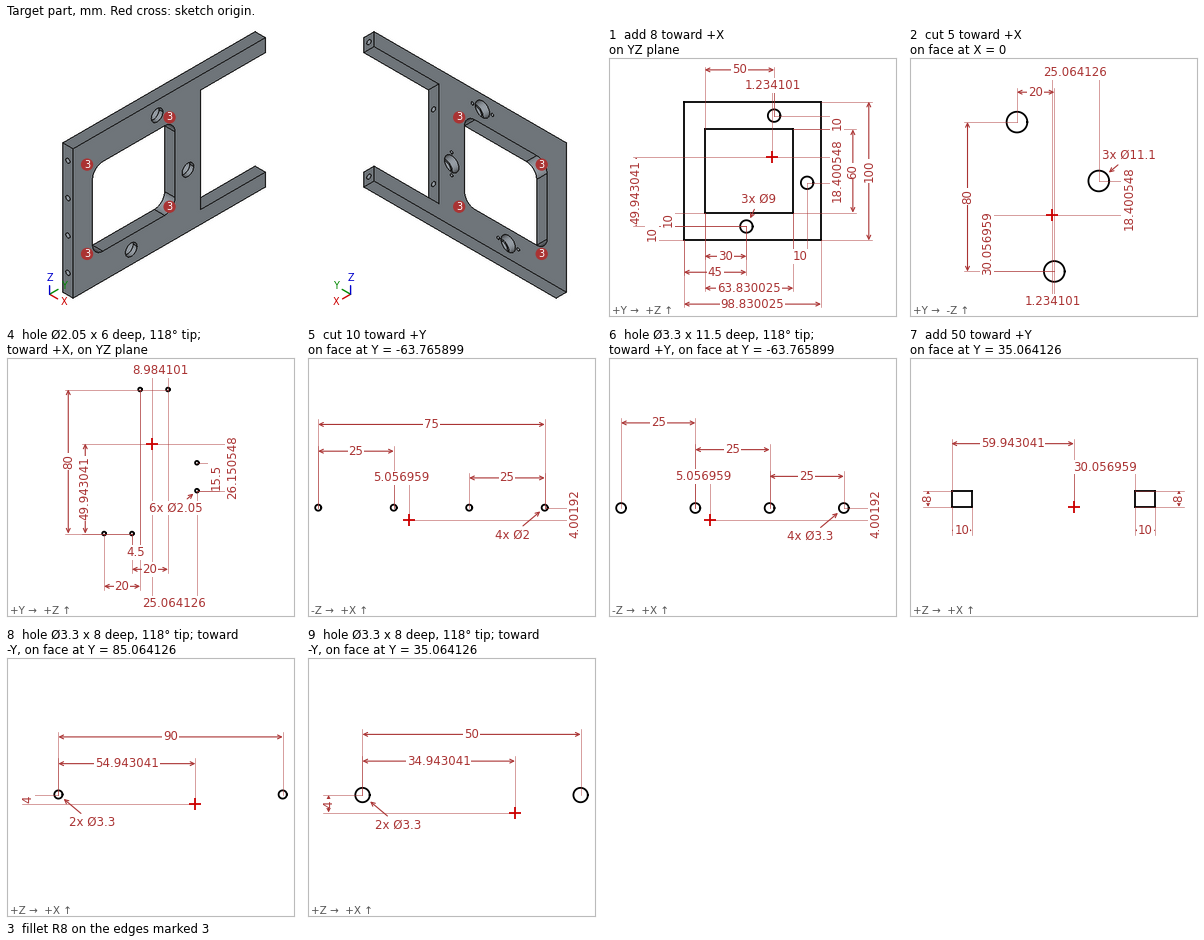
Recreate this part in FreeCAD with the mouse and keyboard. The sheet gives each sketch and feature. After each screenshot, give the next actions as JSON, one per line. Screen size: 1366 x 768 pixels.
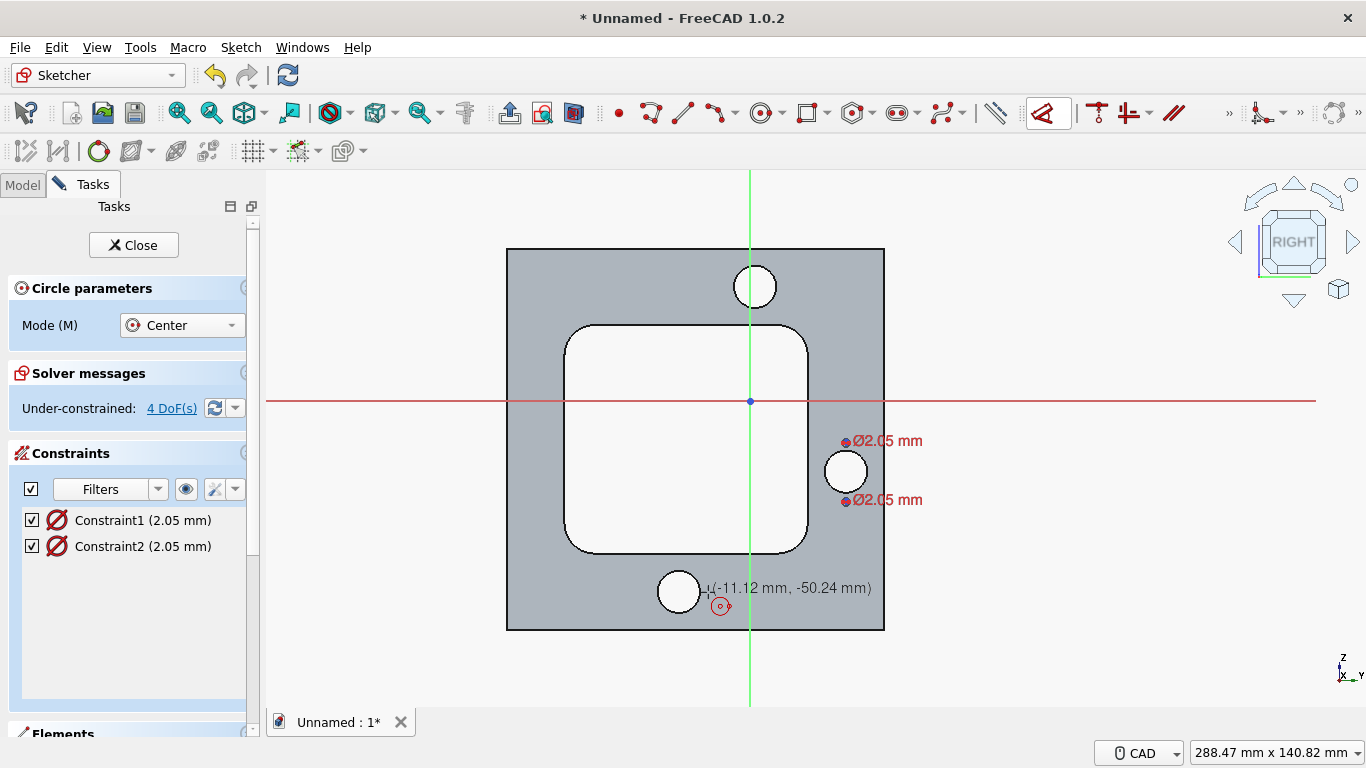
{"action": "left_click", "coordinate": [708, 592]}
{"action": "mouse_move", "coordinate": [711, 589]}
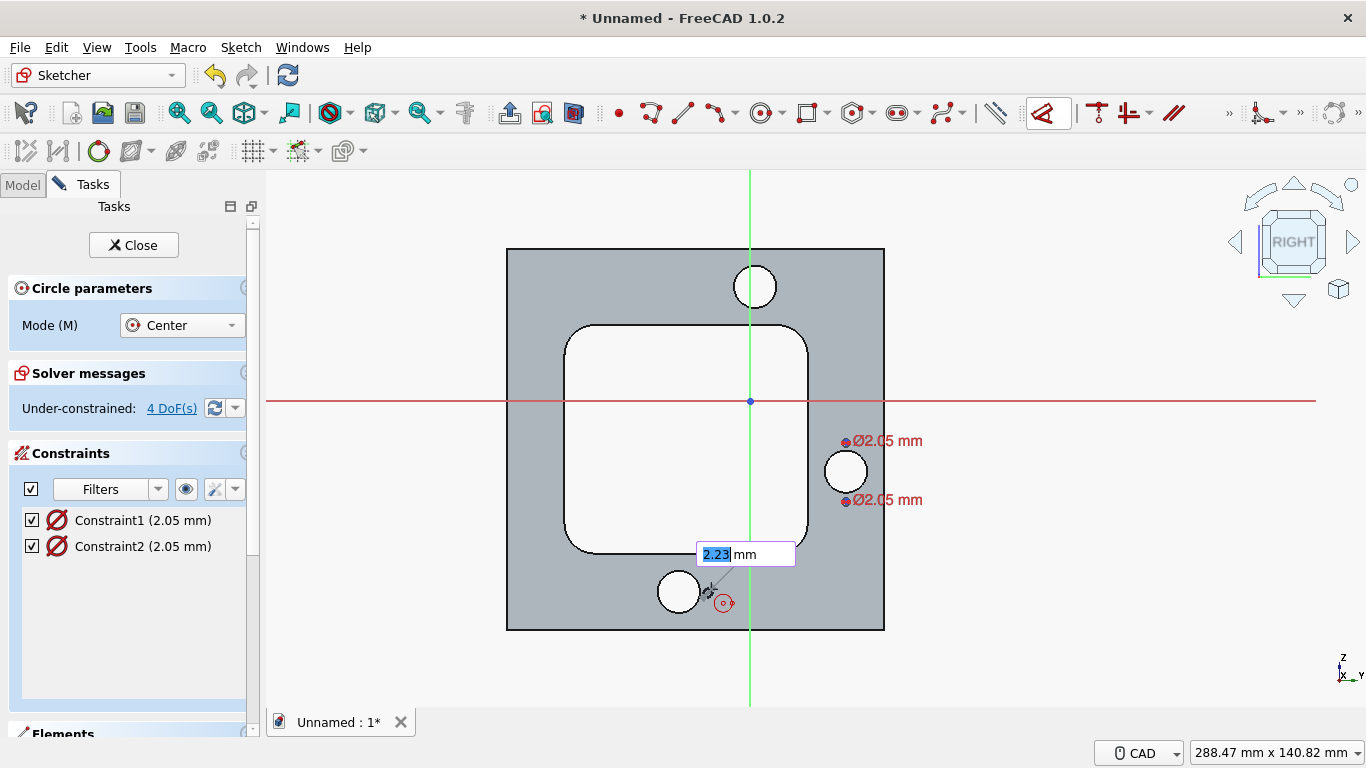
{"action": "type", "text": "2.05"}
{"action": "key", "text": "Return"}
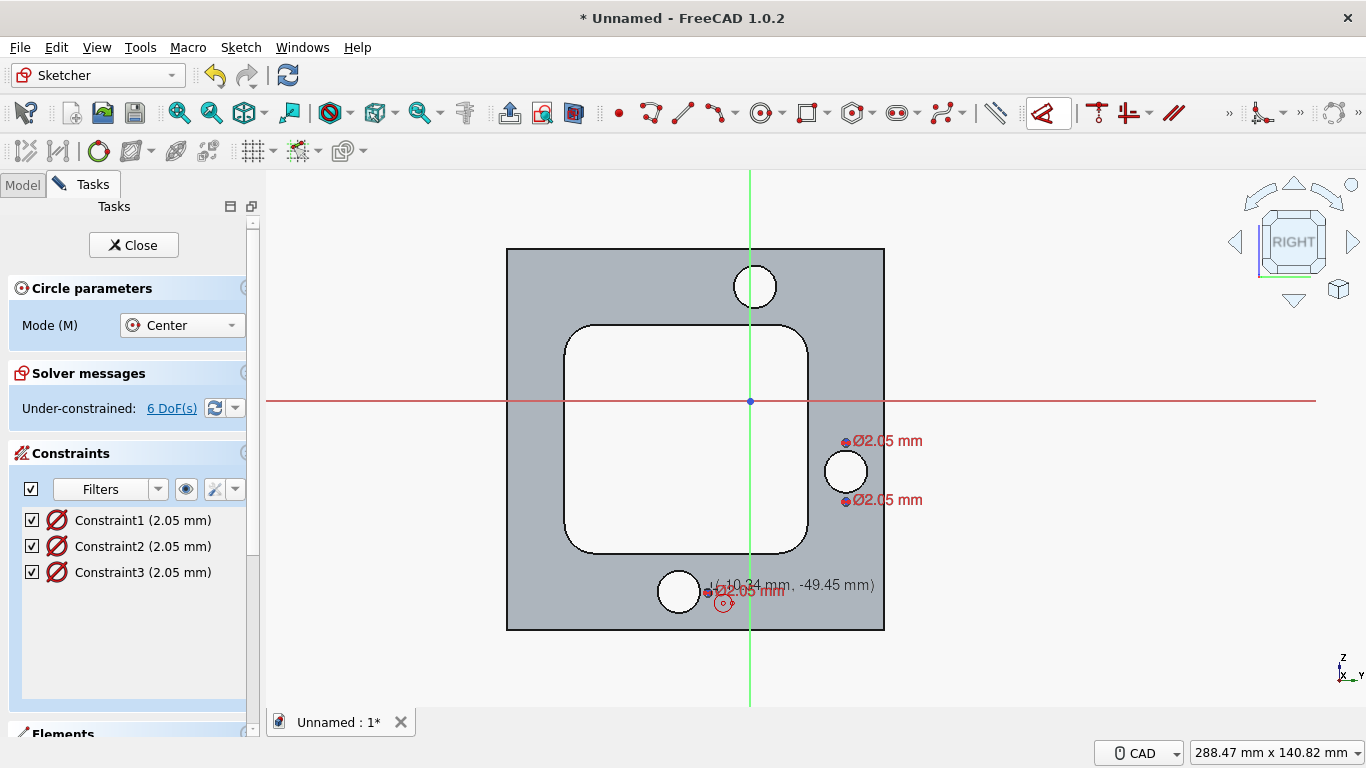
{"action": "scroll", "coordinate": [649, 592], "scroll_direction": "up", "scroll_amount": 9}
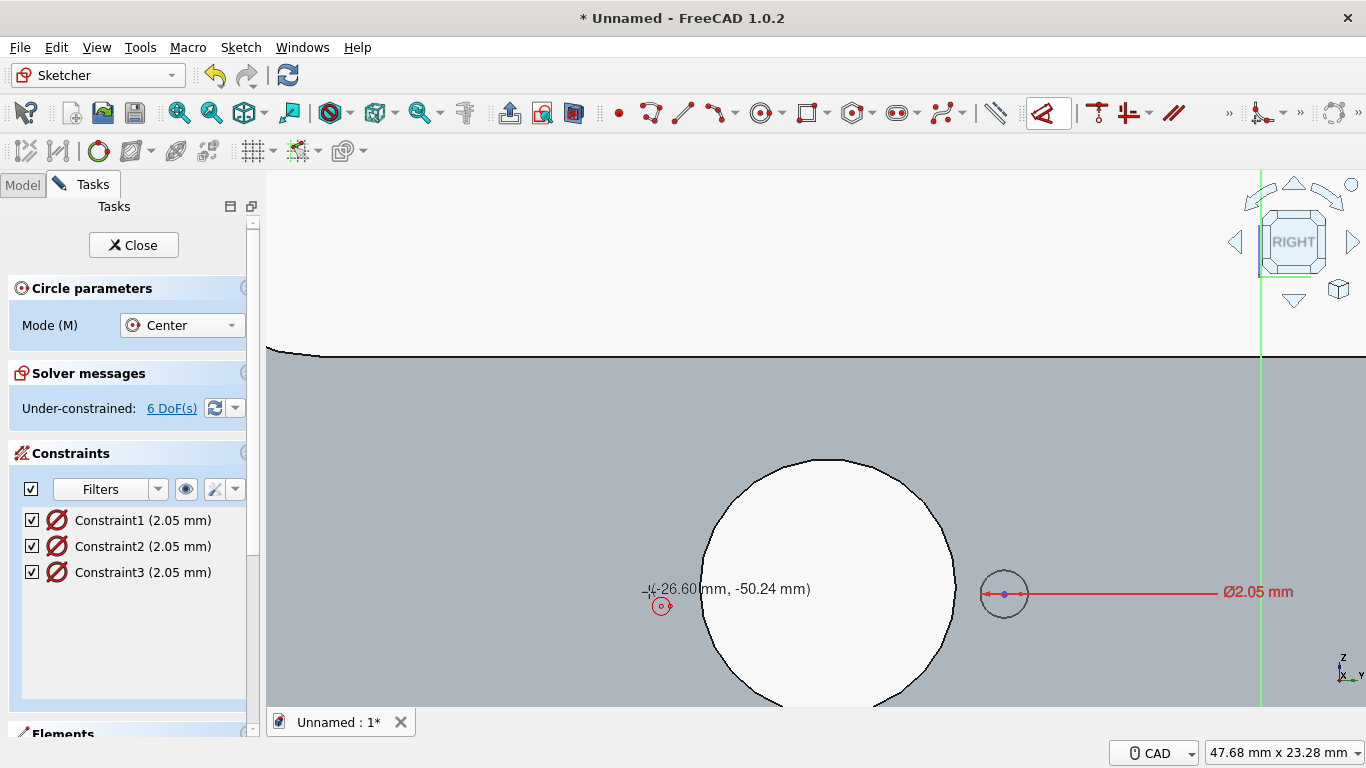
{"action": "scroll", "coordinate": [649, 592], "scroll_direction": "down", "scroll_amount": 9}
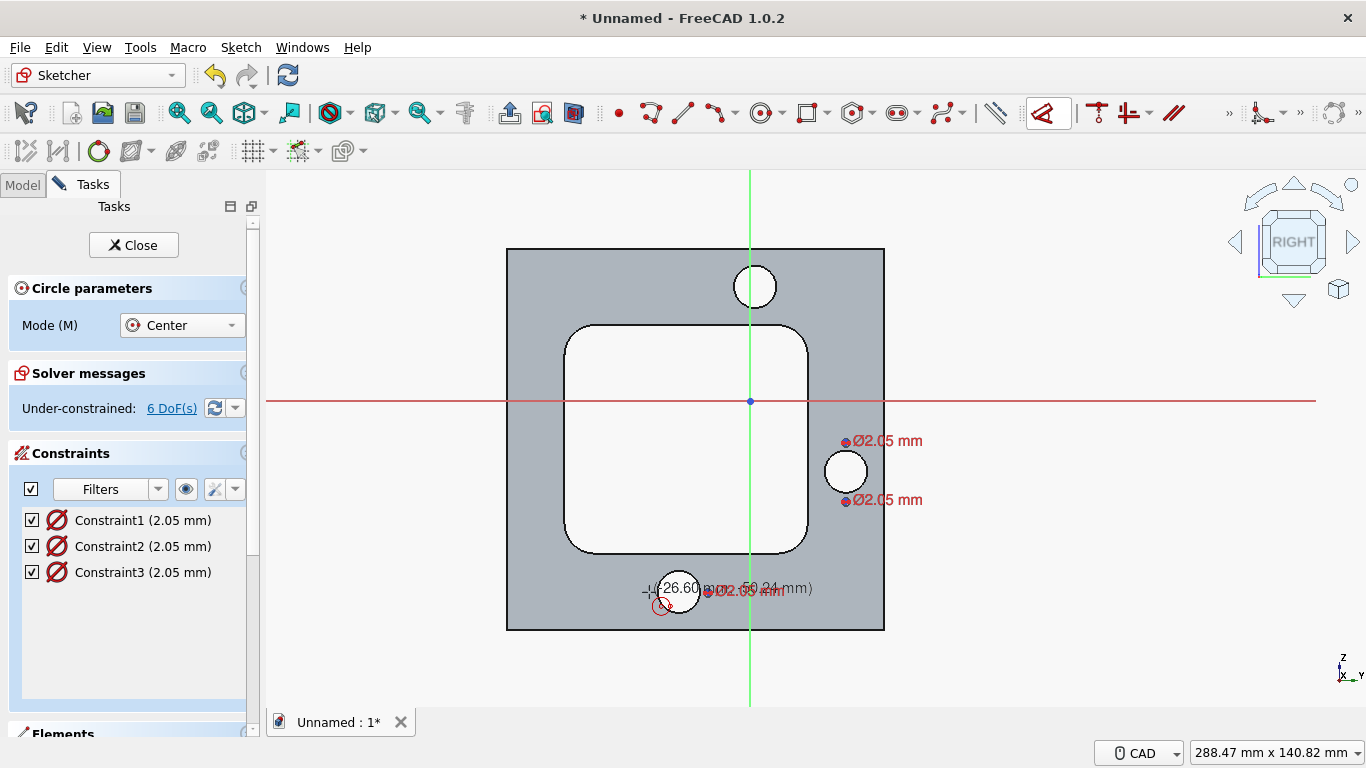
{"action": "left_click", "coordinate": [649, 592]}
{"action": "mouse_move", "coordinate": [652, 589]}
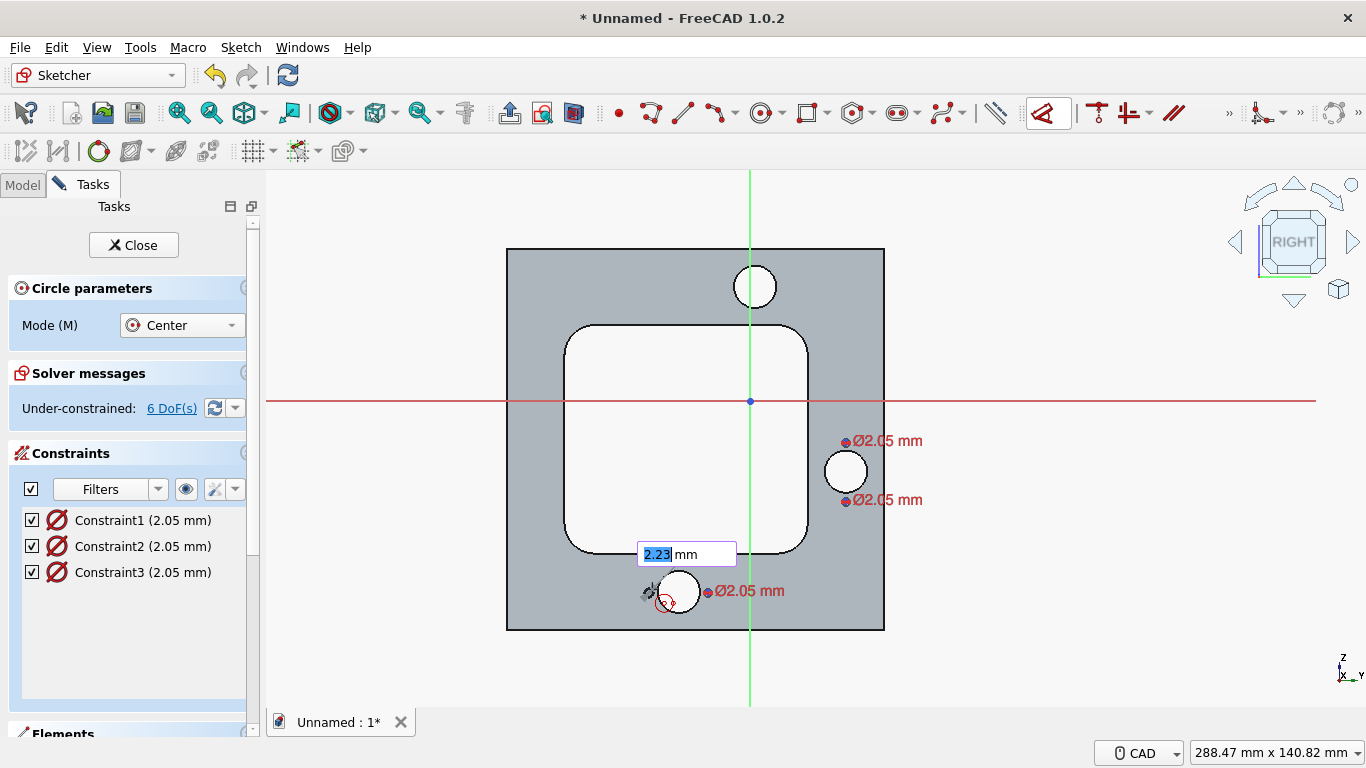
{"action": "type", "text": "2.05"}
{"action": "key", "text": "Return"}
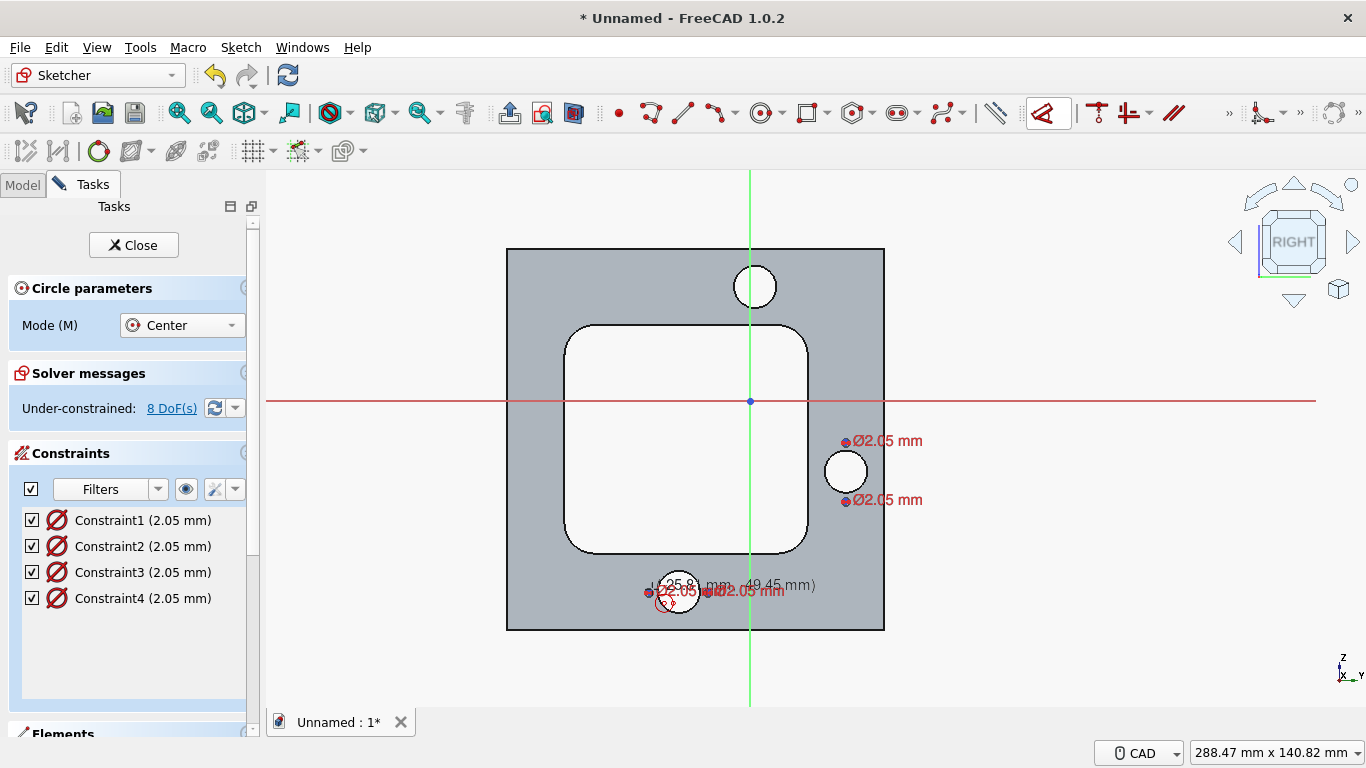
{"action": "scroll", "coordinate": [785, 287], "scroll_direction": "up", "scroll_amount": 9}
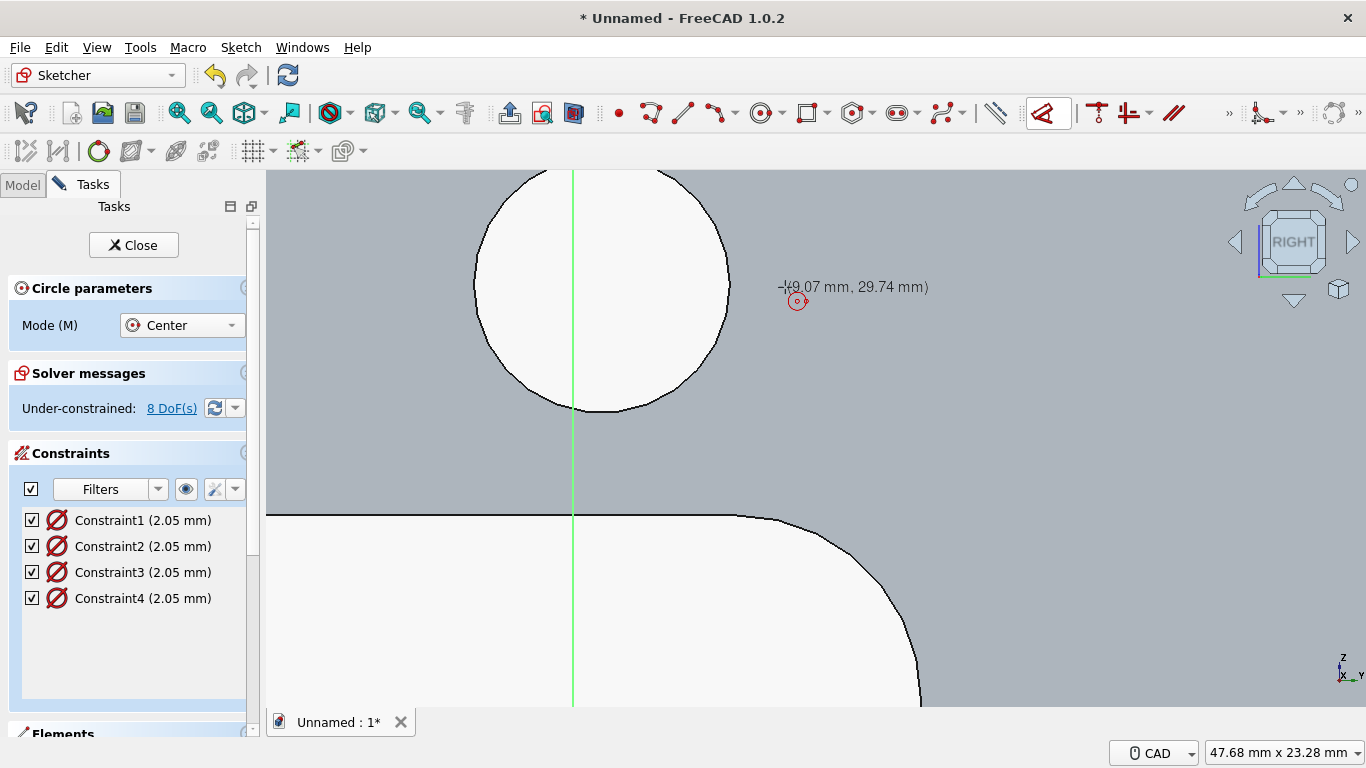
{"action": "scroll", "coordinate": [785, 286], "scroll_direction": "down", "scroll_amount": 9}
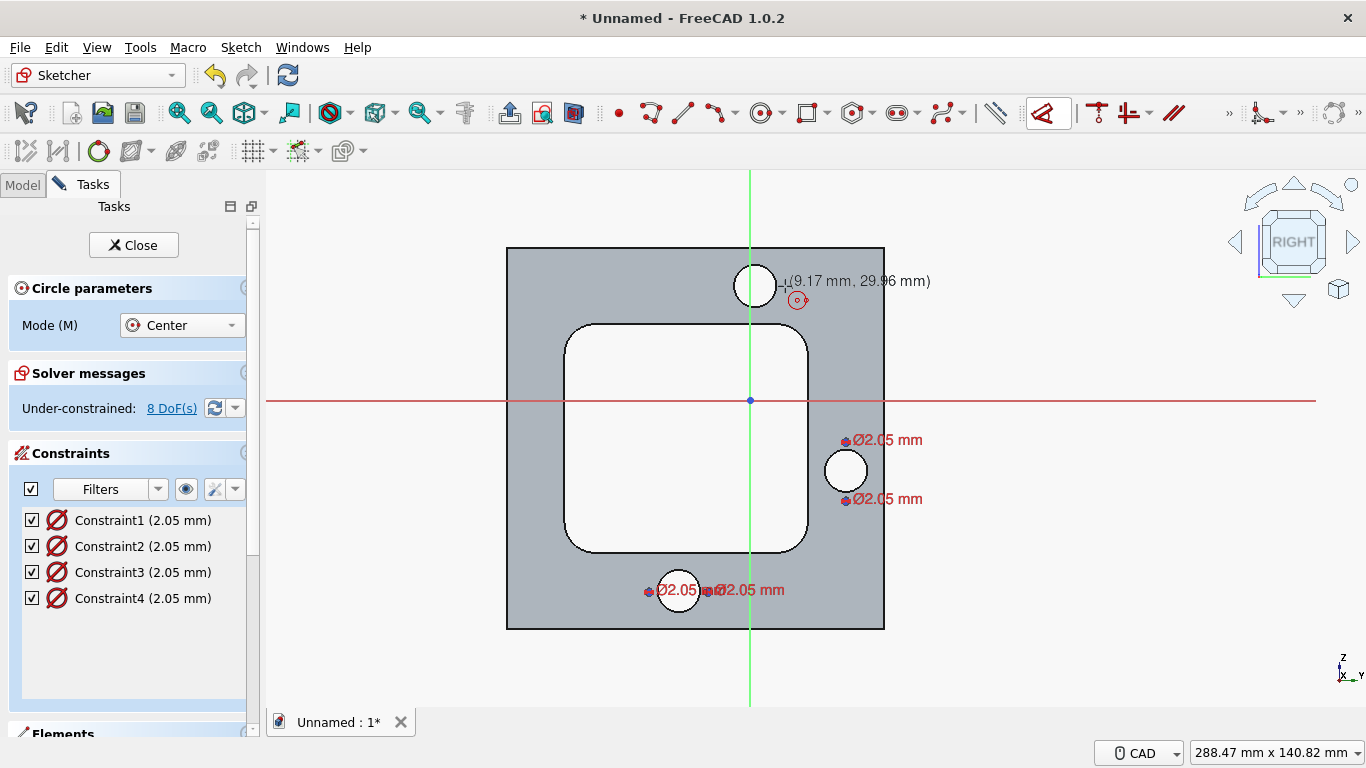
{"action": "left_click", "coordinate": [785, 286]}
{"action": "mouse_move", "coordinate": [787, 283]}